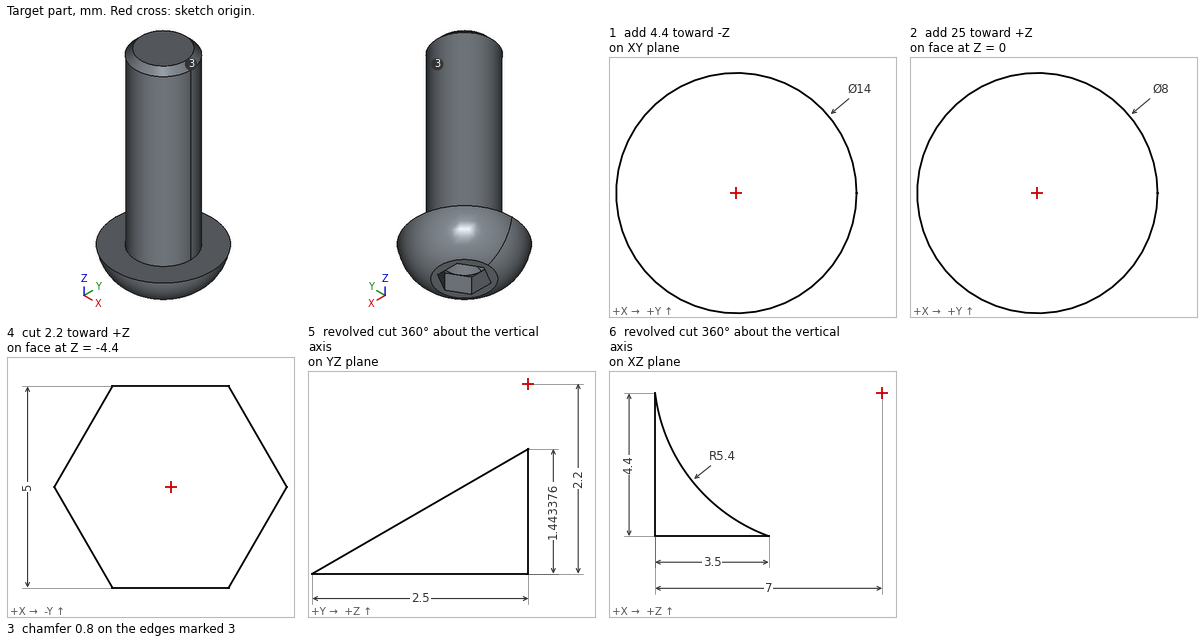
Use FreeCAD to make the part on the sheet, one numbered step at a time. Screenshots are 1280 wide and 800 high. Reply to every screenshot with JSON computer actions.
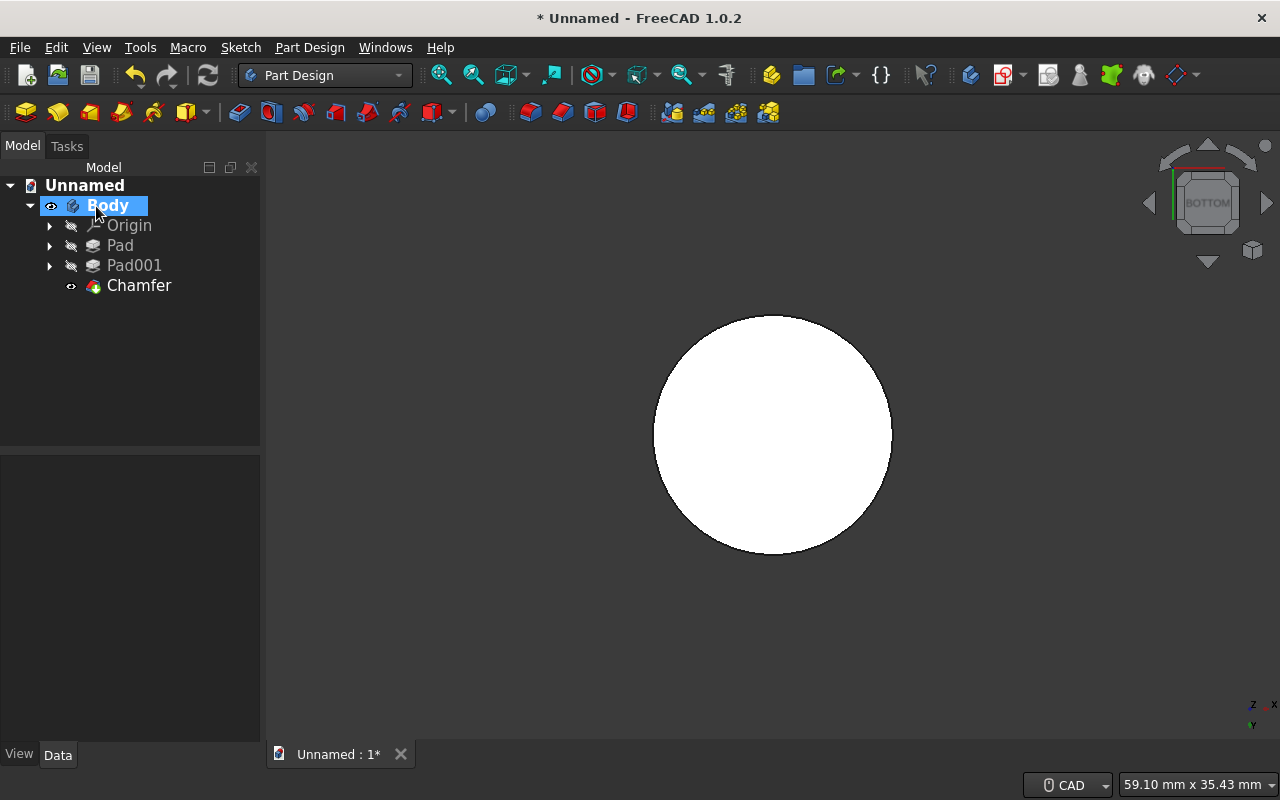
{"action": "left_click", "coordinate": [442, 76]}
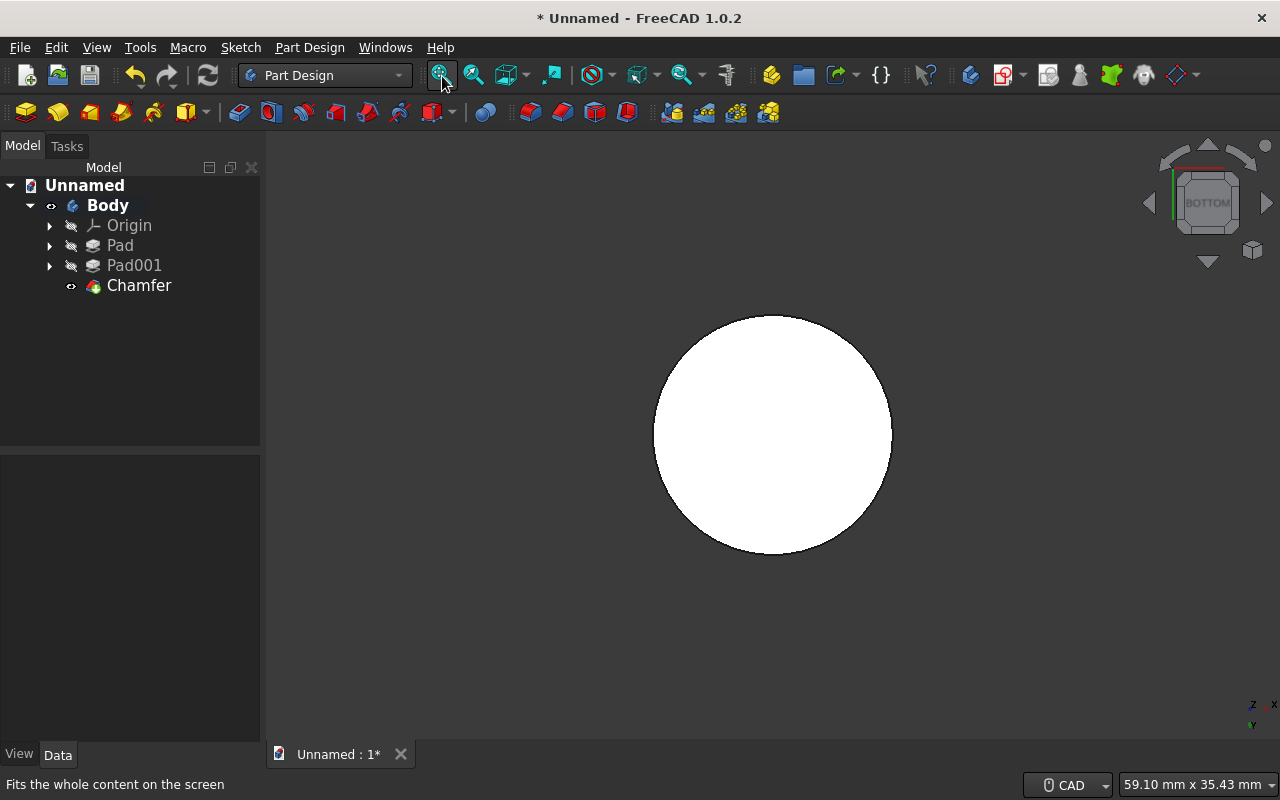
{"action": "left_click", "coordinate": [773, 434]}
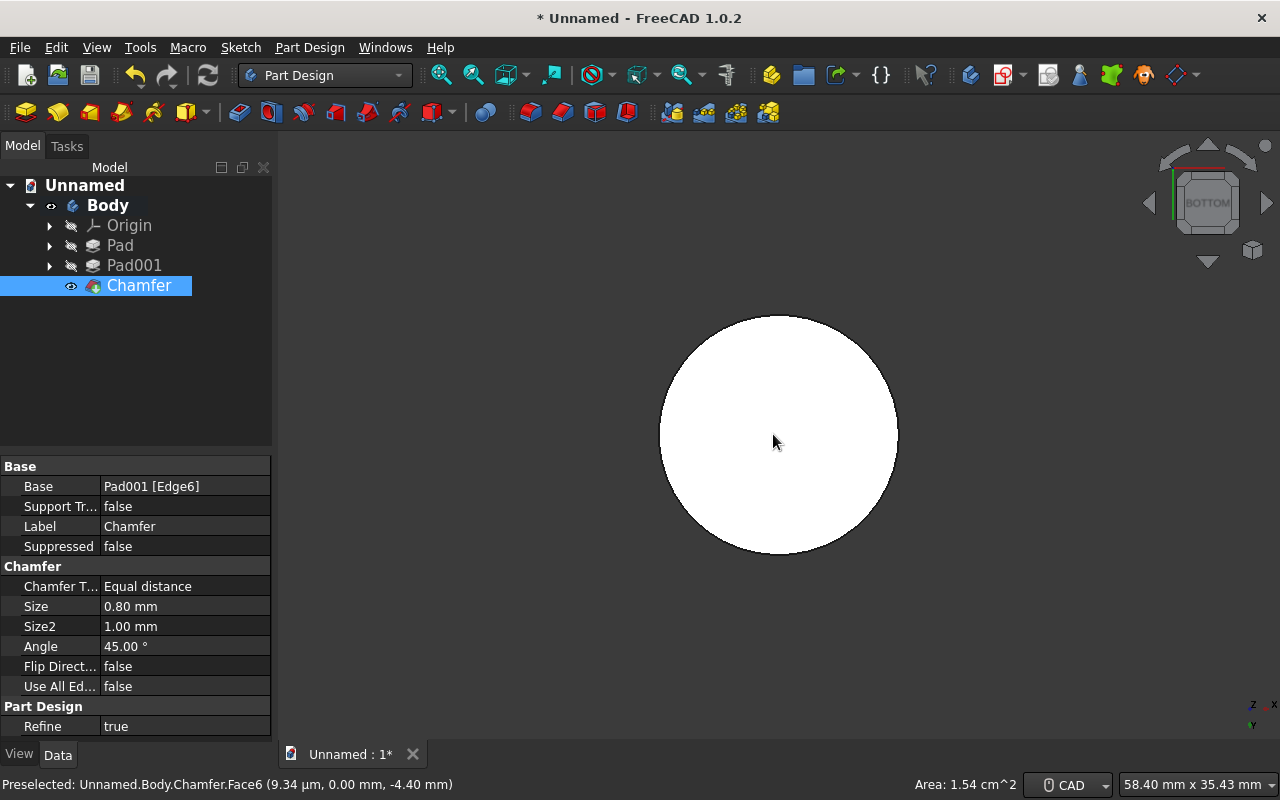
{"action": "left_click", "coordinate": [1004, 76]}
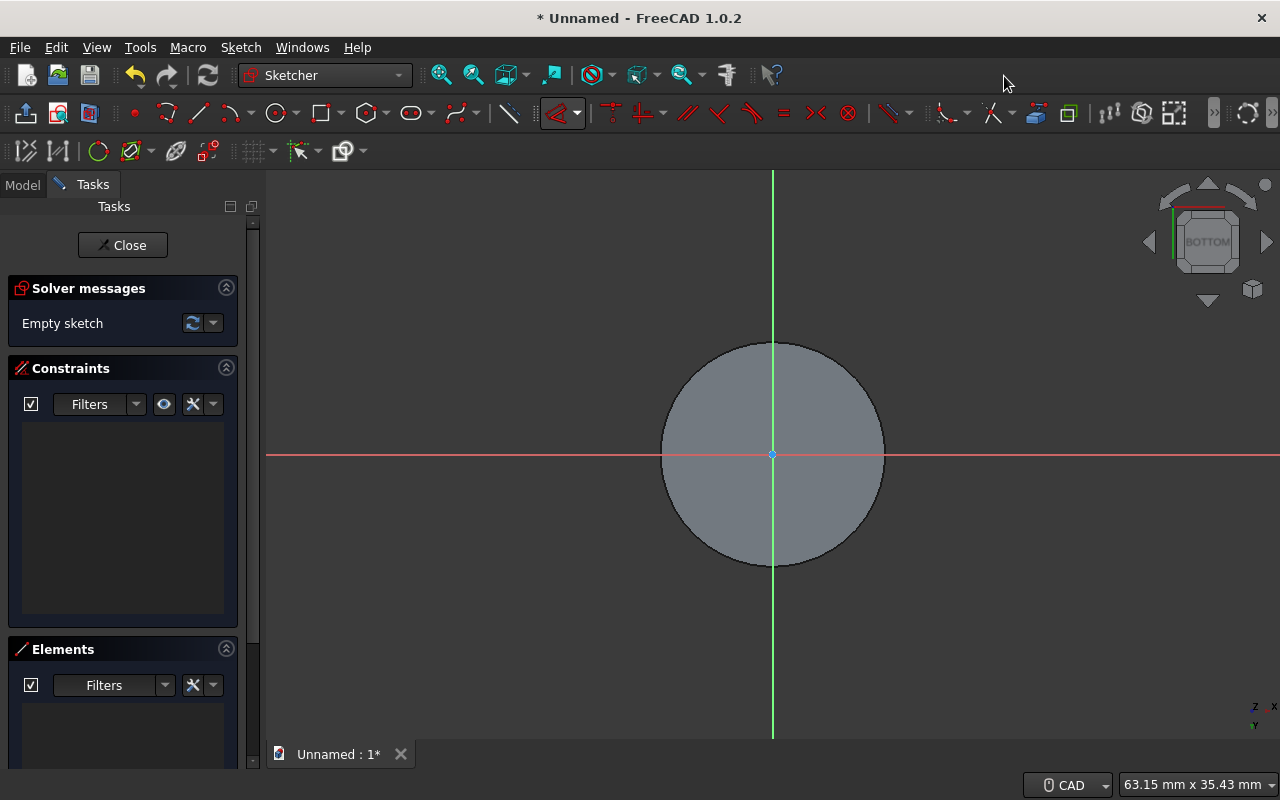
{"action": "scroll", "coordinate": [790, 454], "scroll_direction": "up", "scroll_amount": 8}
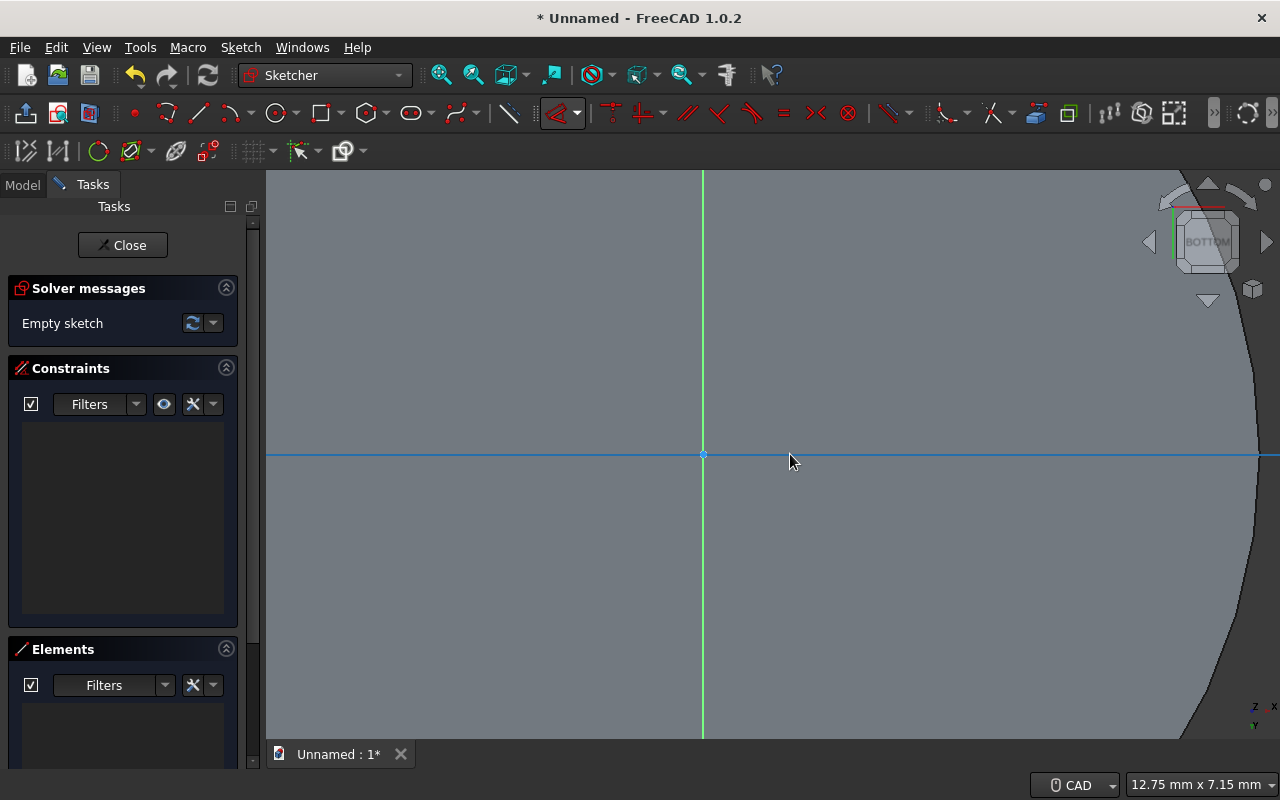
{"action": "left_click", "coordinate": [366, 114]}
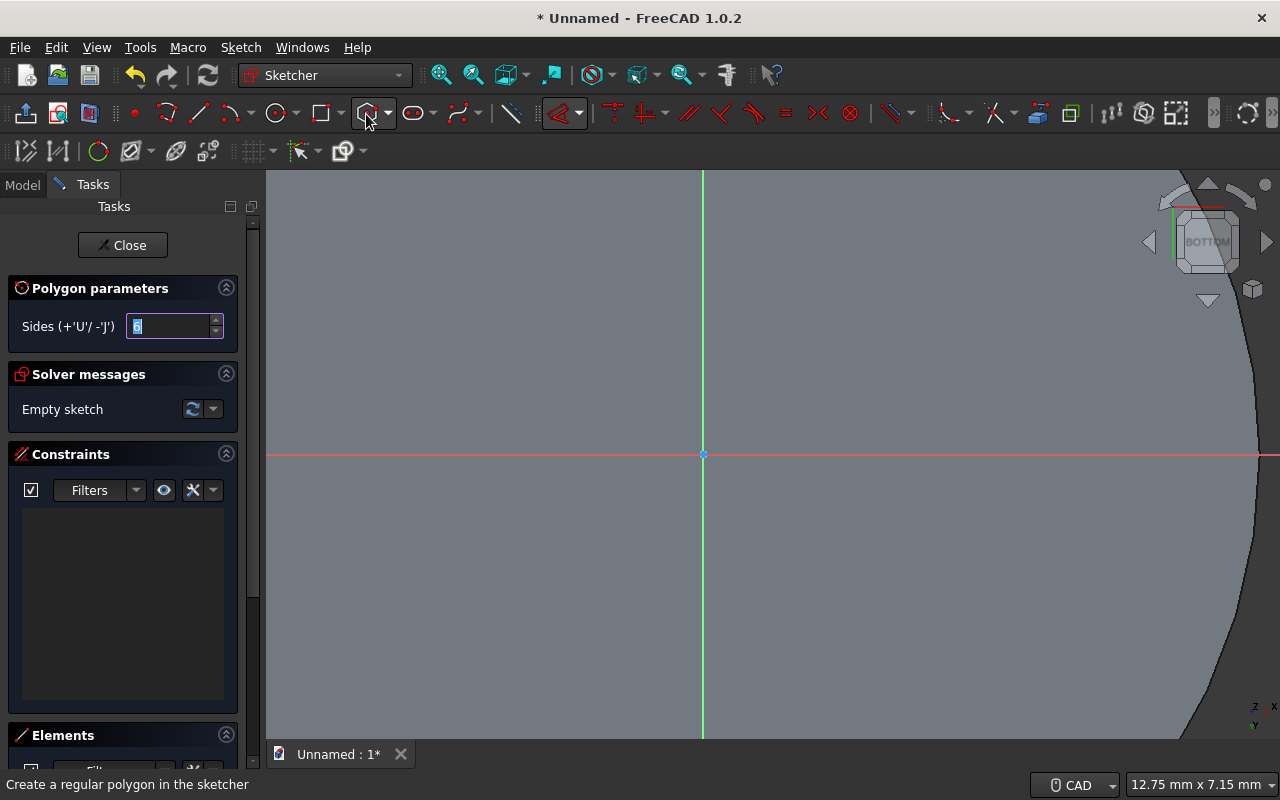
{"action": "left_click", "coordinate": [703, 454]}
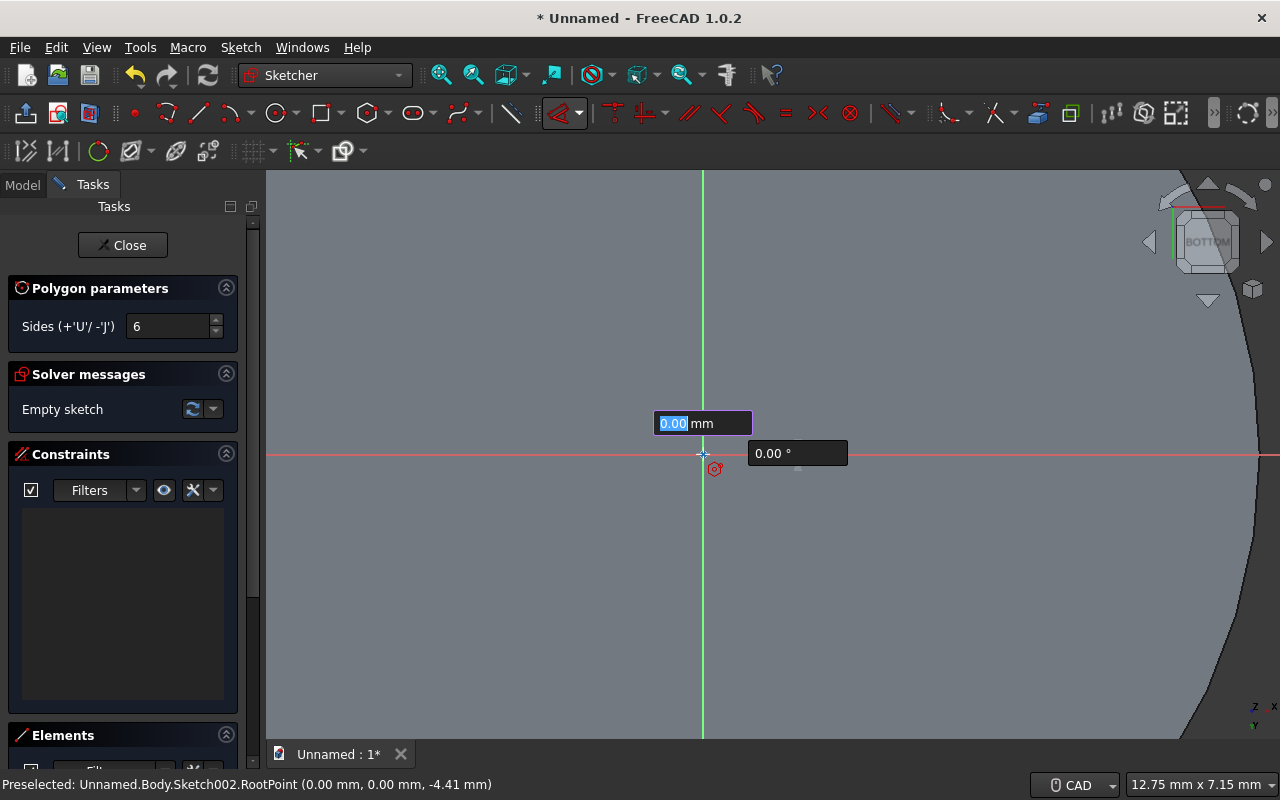
{"action": "left_click", "coordinate": [473, 454]}
{"action": "right_click", "coordinate": [473, 454]}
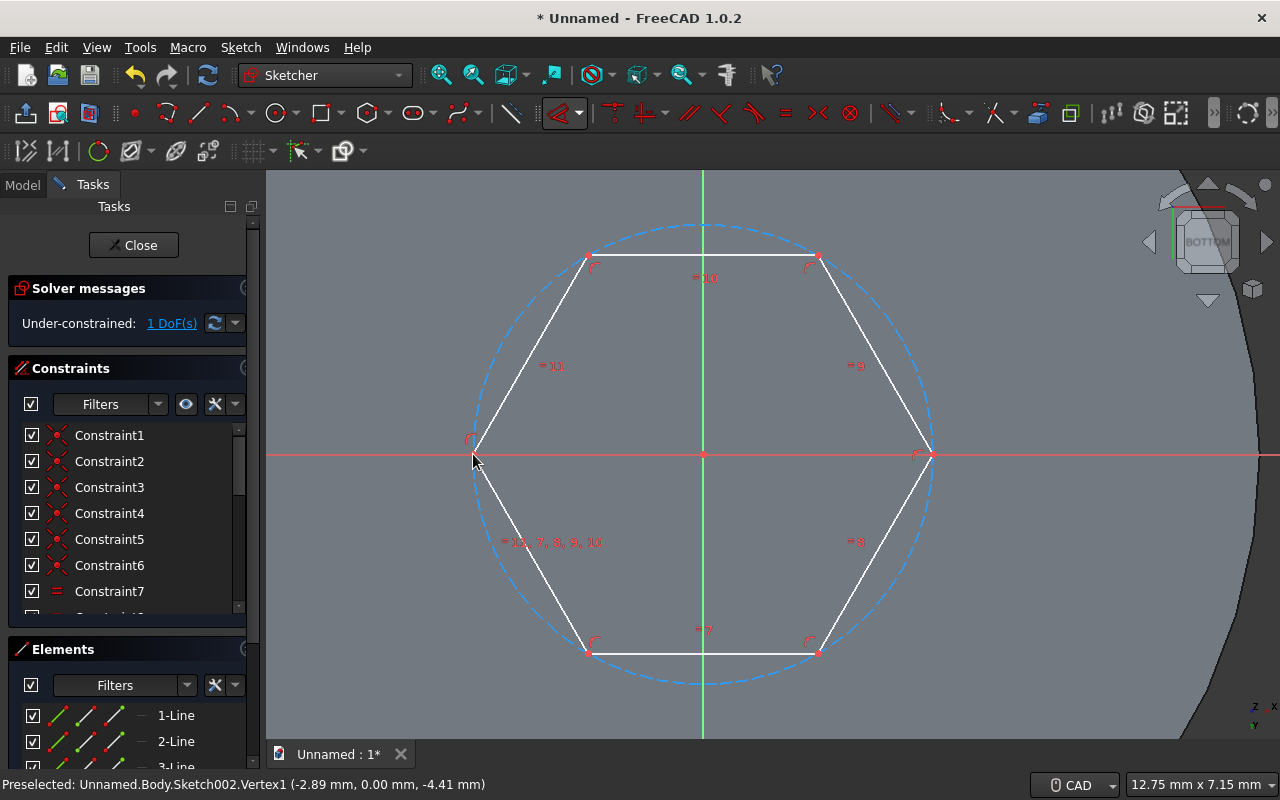
{"action": "left_click", "coordinate": [588, 654]}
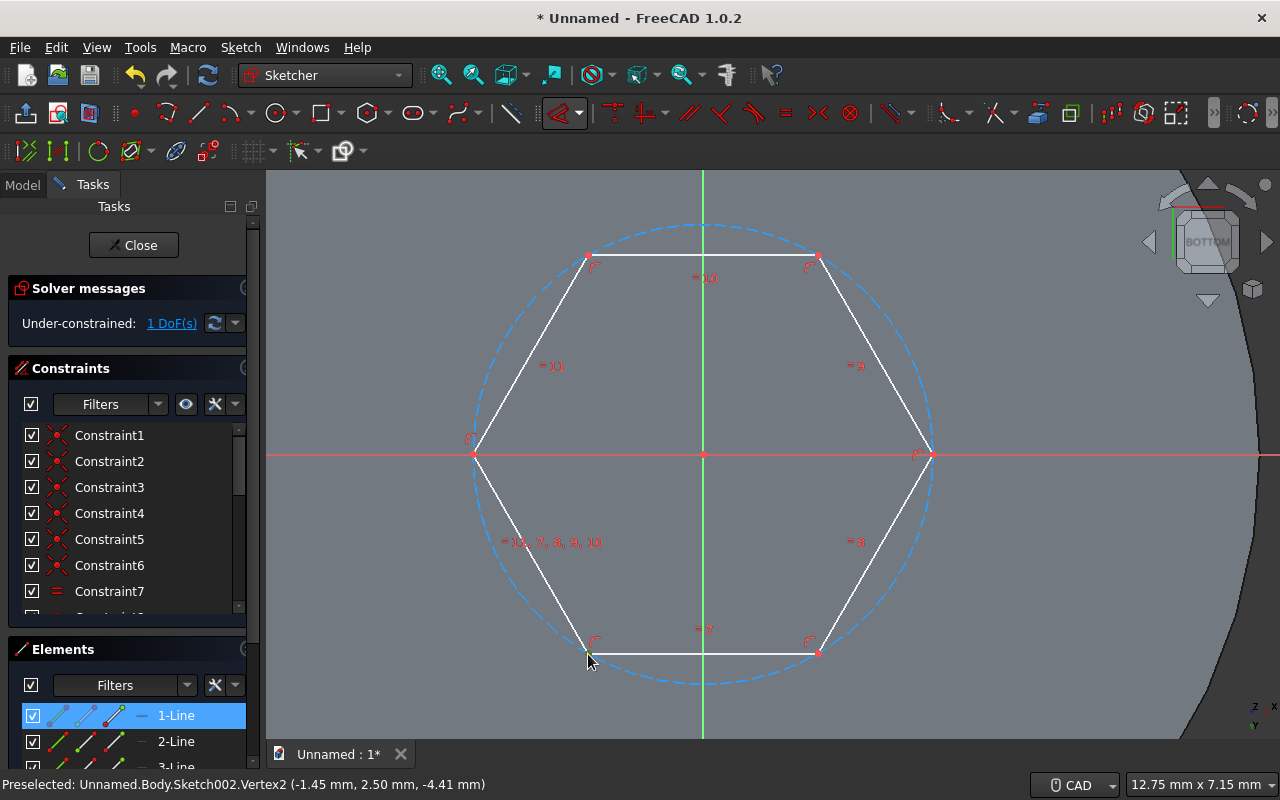
{"action": "left_click", "coordinate": [818, 255]}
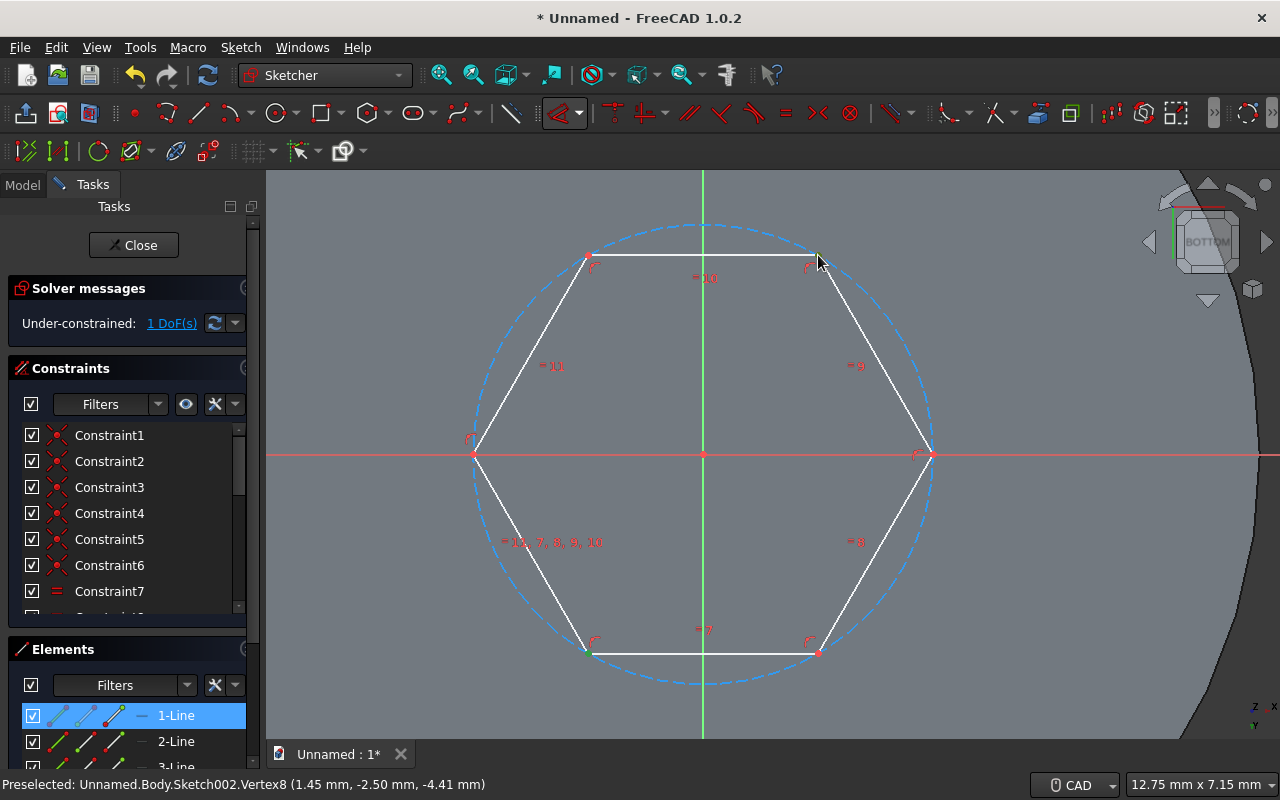
{"action": "key", "text": "i"}